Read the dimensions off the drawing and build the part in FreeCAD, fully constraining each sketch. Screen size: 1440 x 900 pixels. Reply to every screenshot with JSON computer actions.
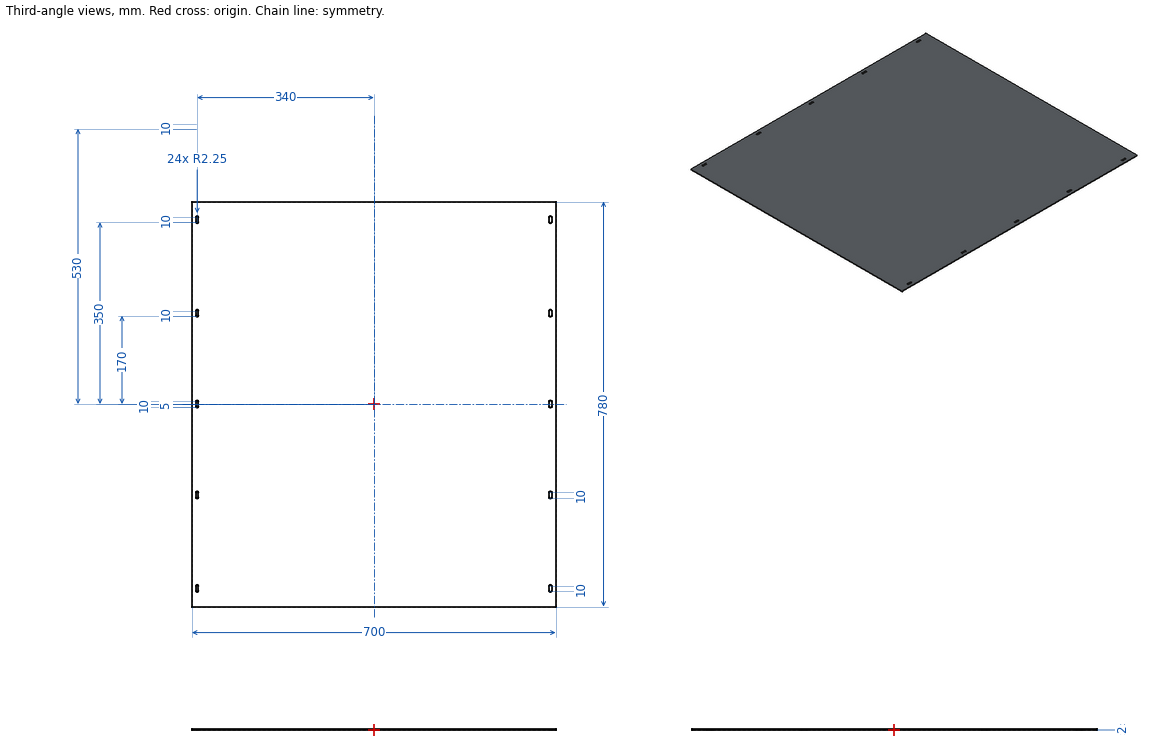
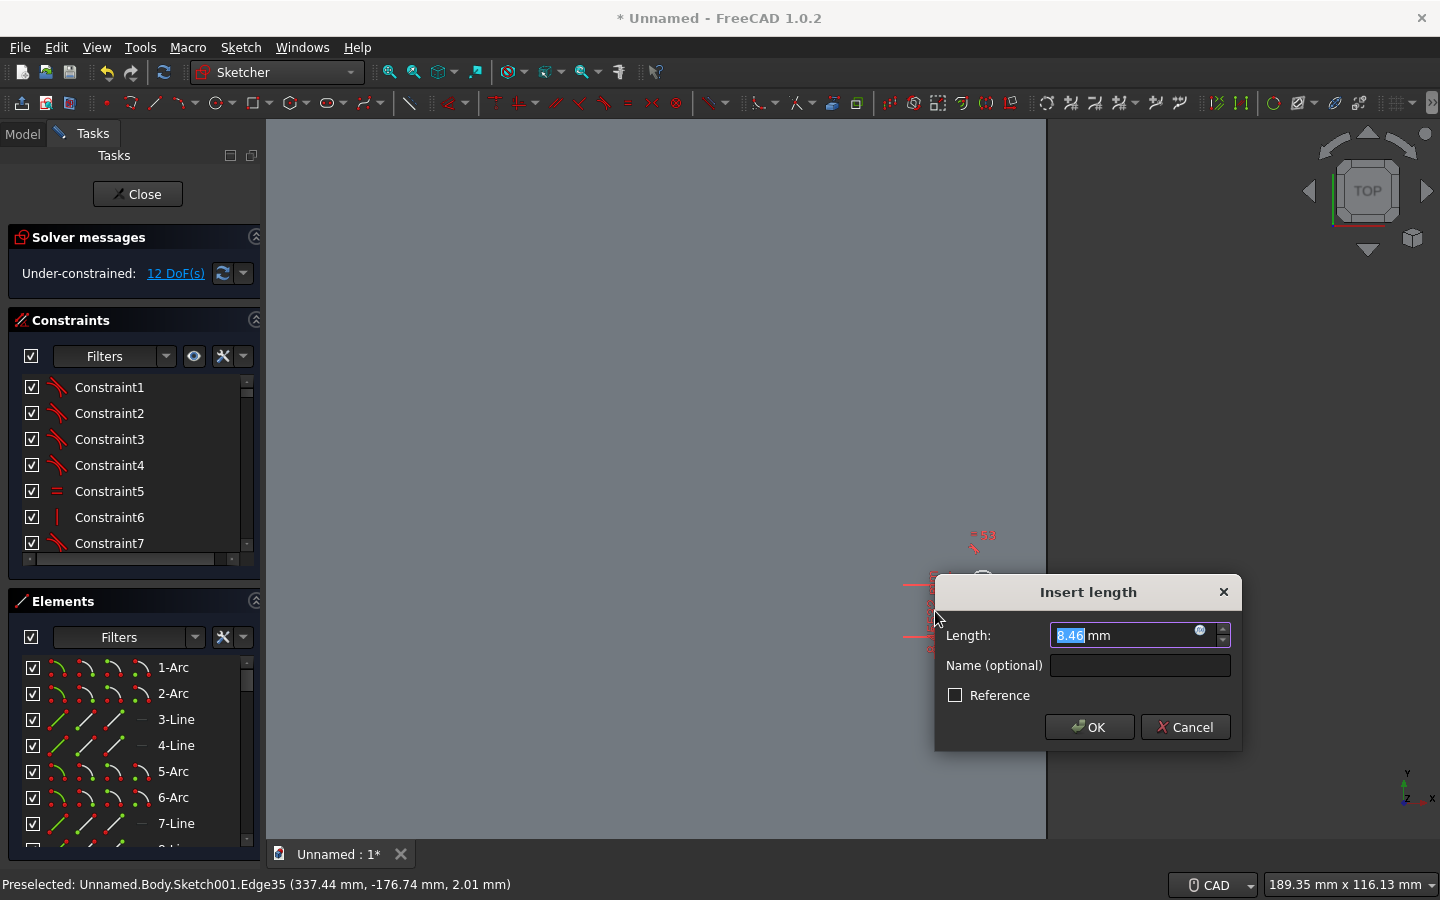
{"action": "type", "text": "10"}
{"action": "key", "text": "Return"}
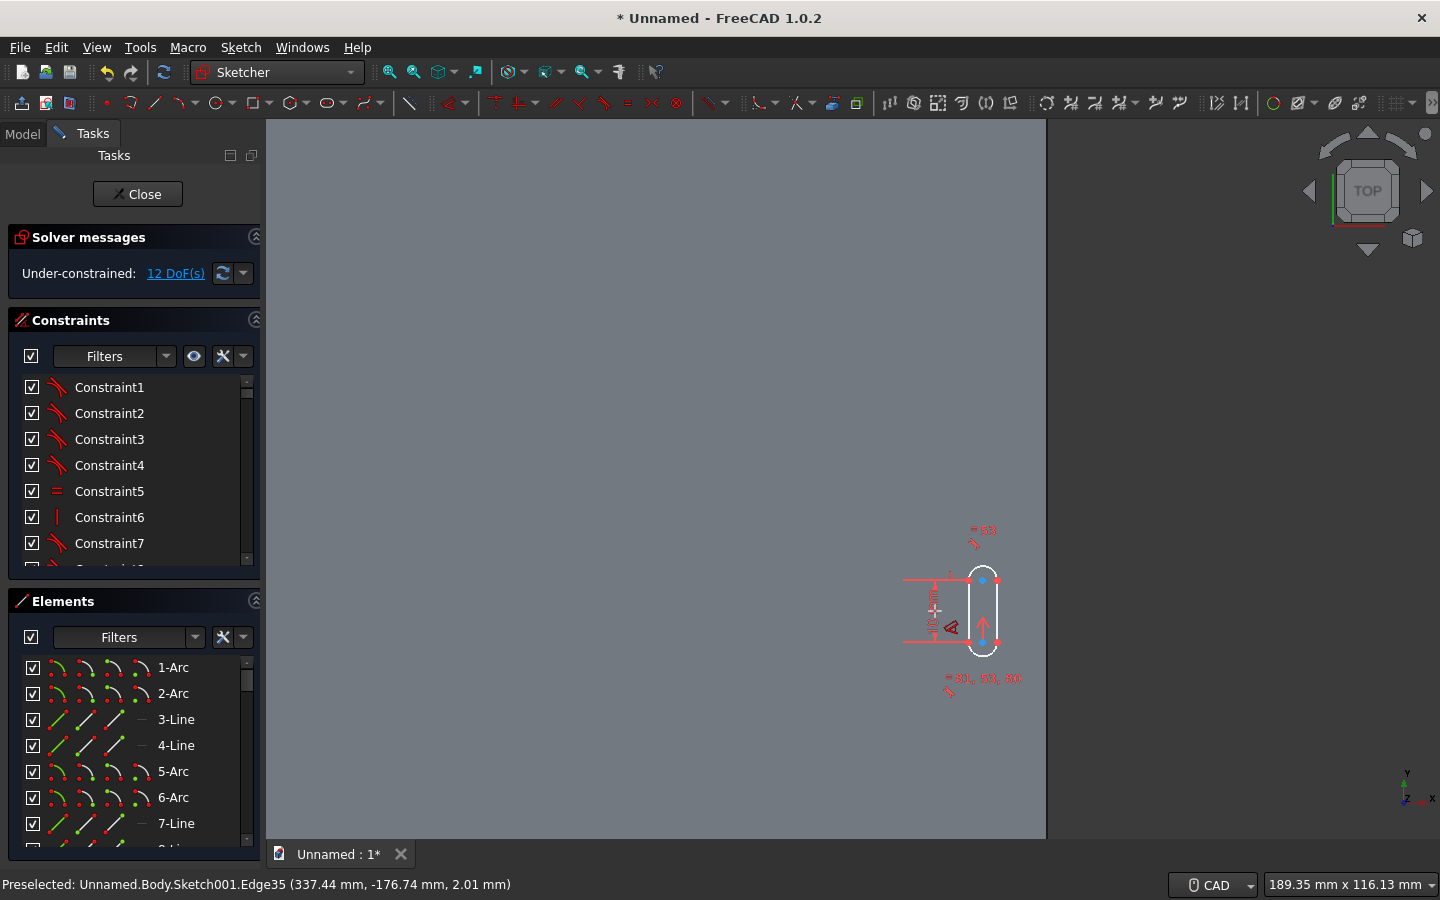
{"action": "scroll", "coordinate": [975, 630], "scroll_direction": "down", "scroll_amount": 12}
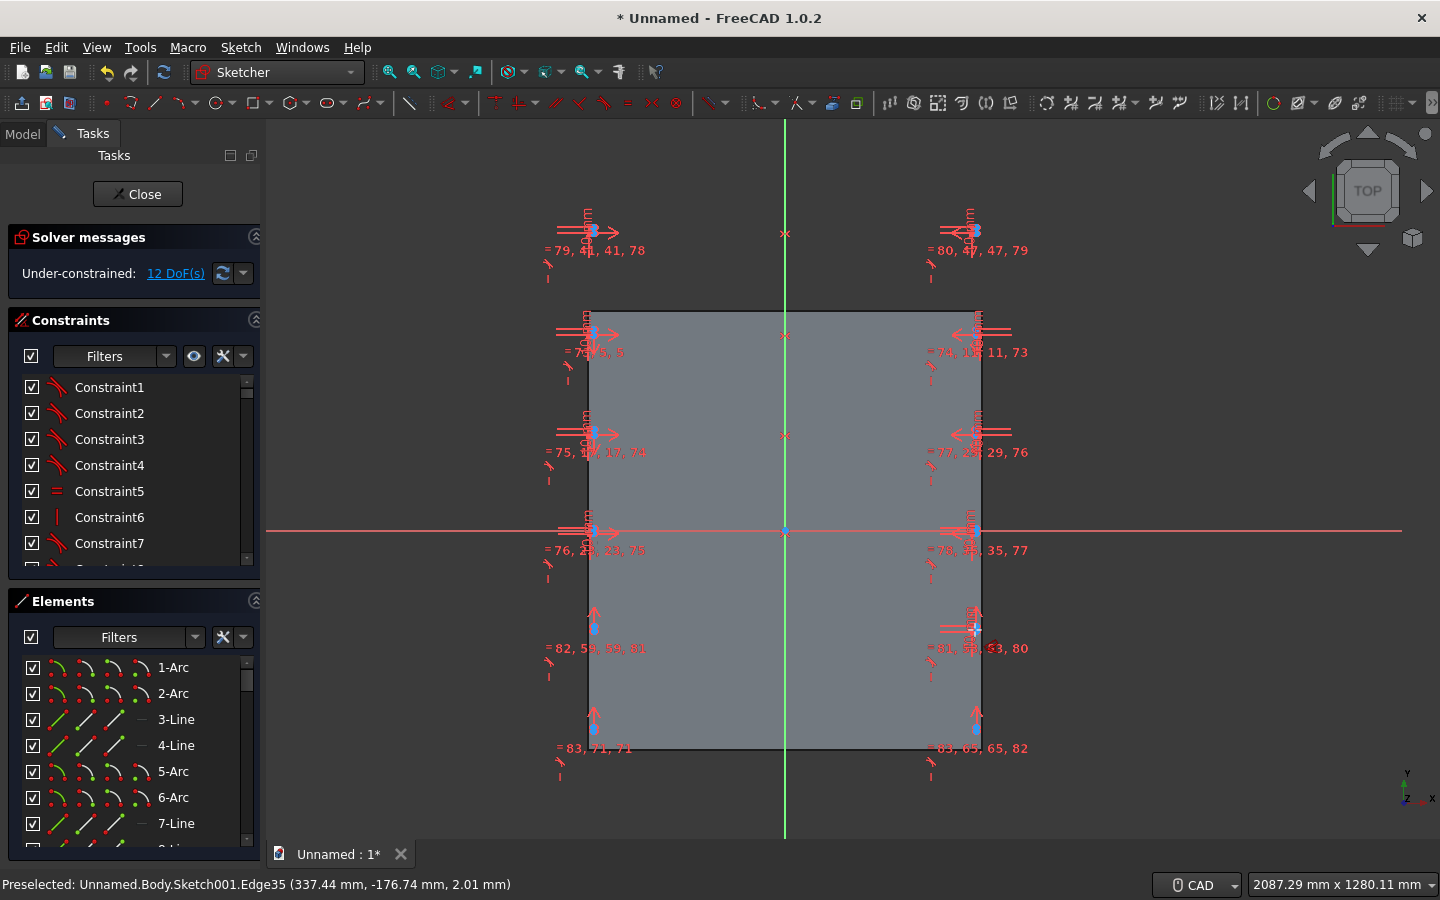
{"action": "scroll", "coordinate": [593, 630], "scroll_direction": "up", "scroll_amount": 11}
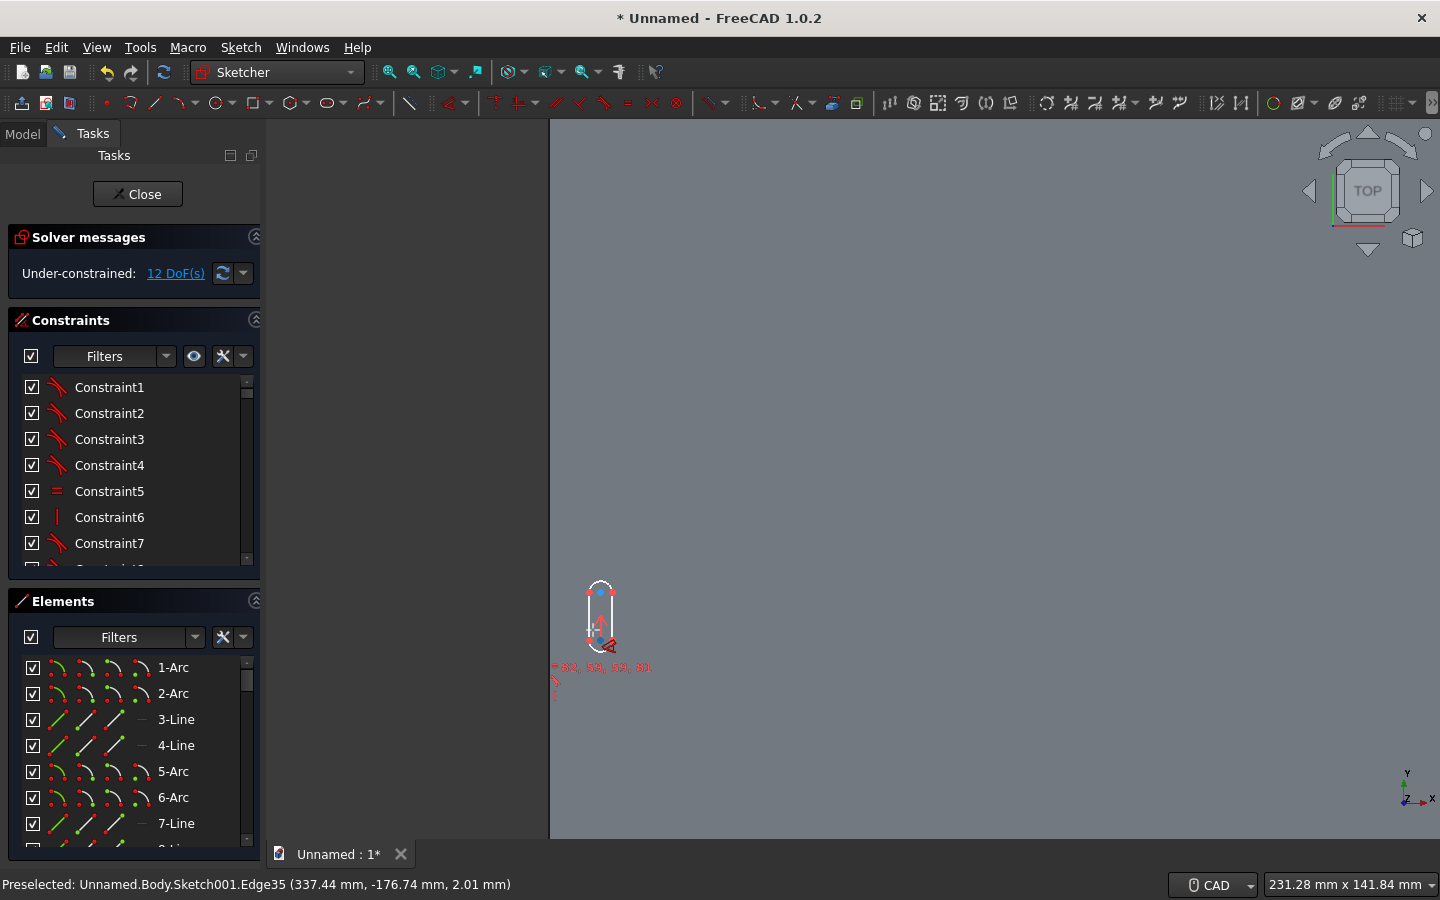
{"action": "left_click", "coordinate": [589, 626]}
{"action": "left_click", "coordinate": [555, 617]}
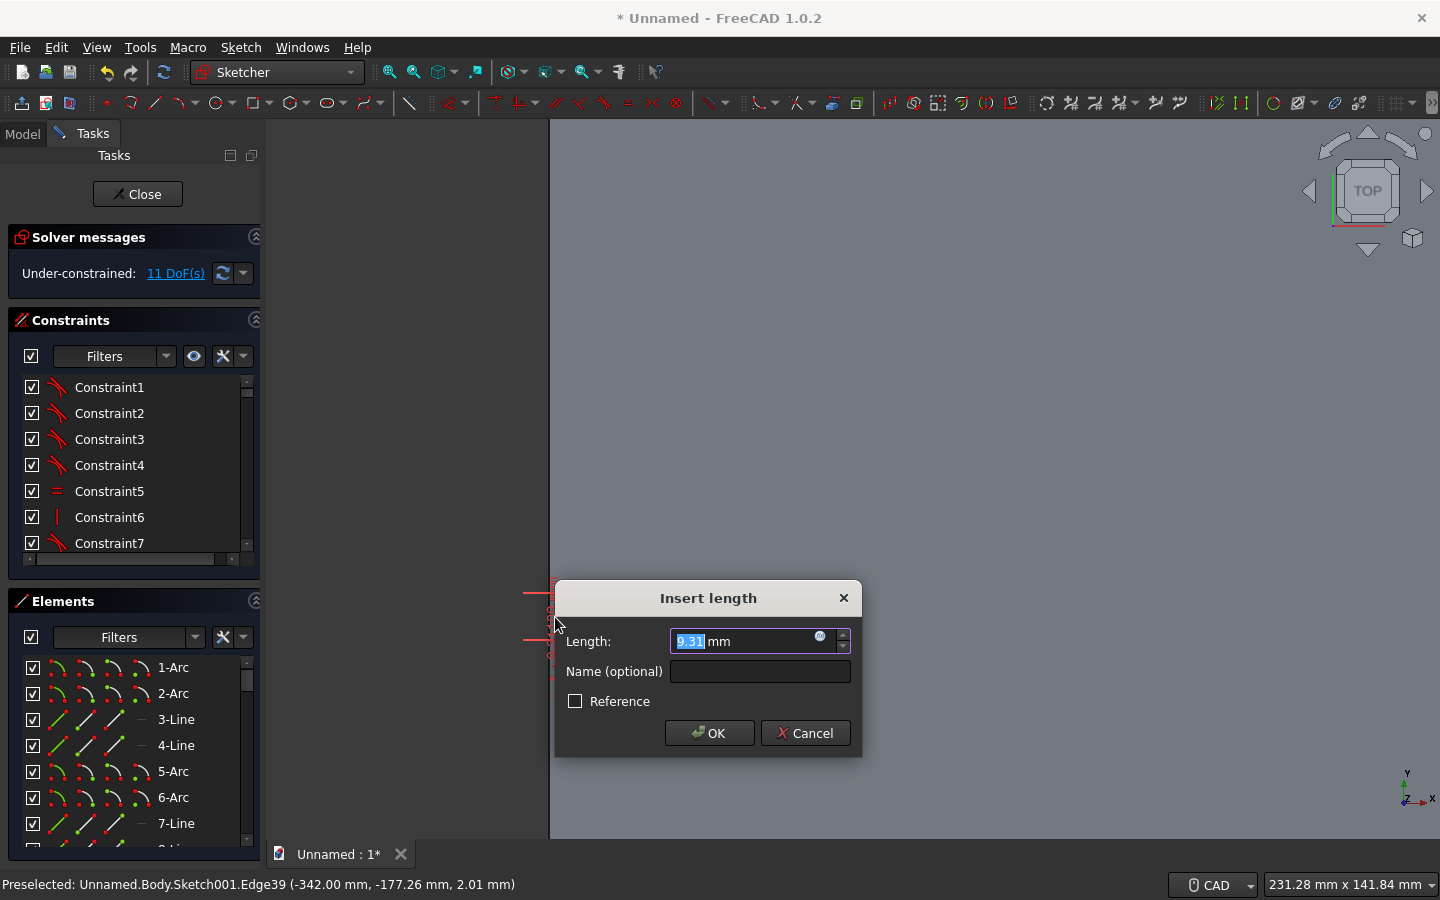
{"action": "type", "text": "10"}
{"action": "key", "text": "Return"}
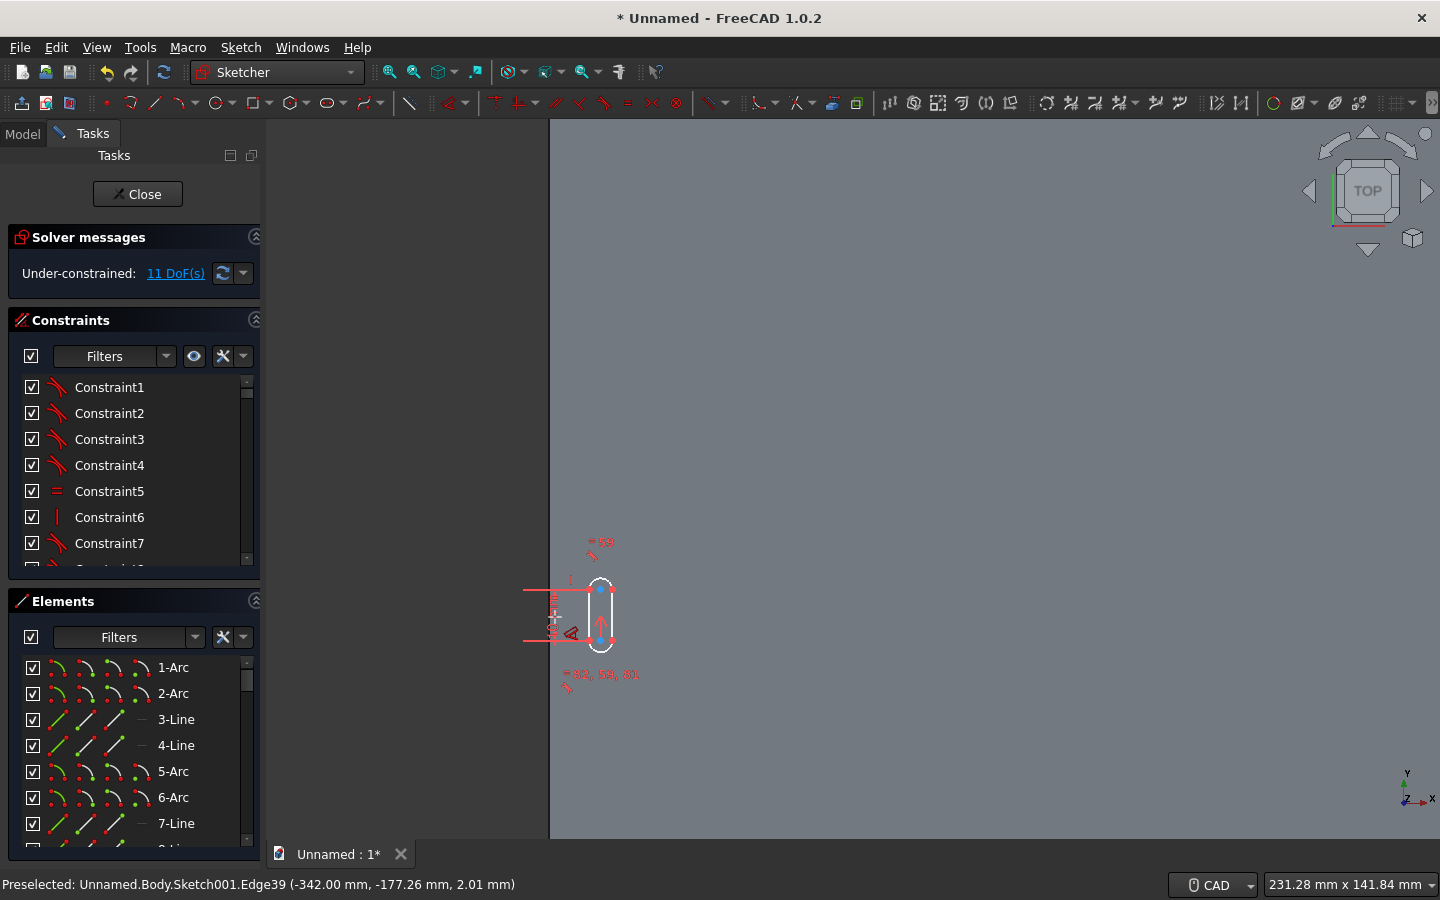
{"action": "scroll", "coordinate": [593, 630], "scroll_direction": "down", "scroll_amount": 11}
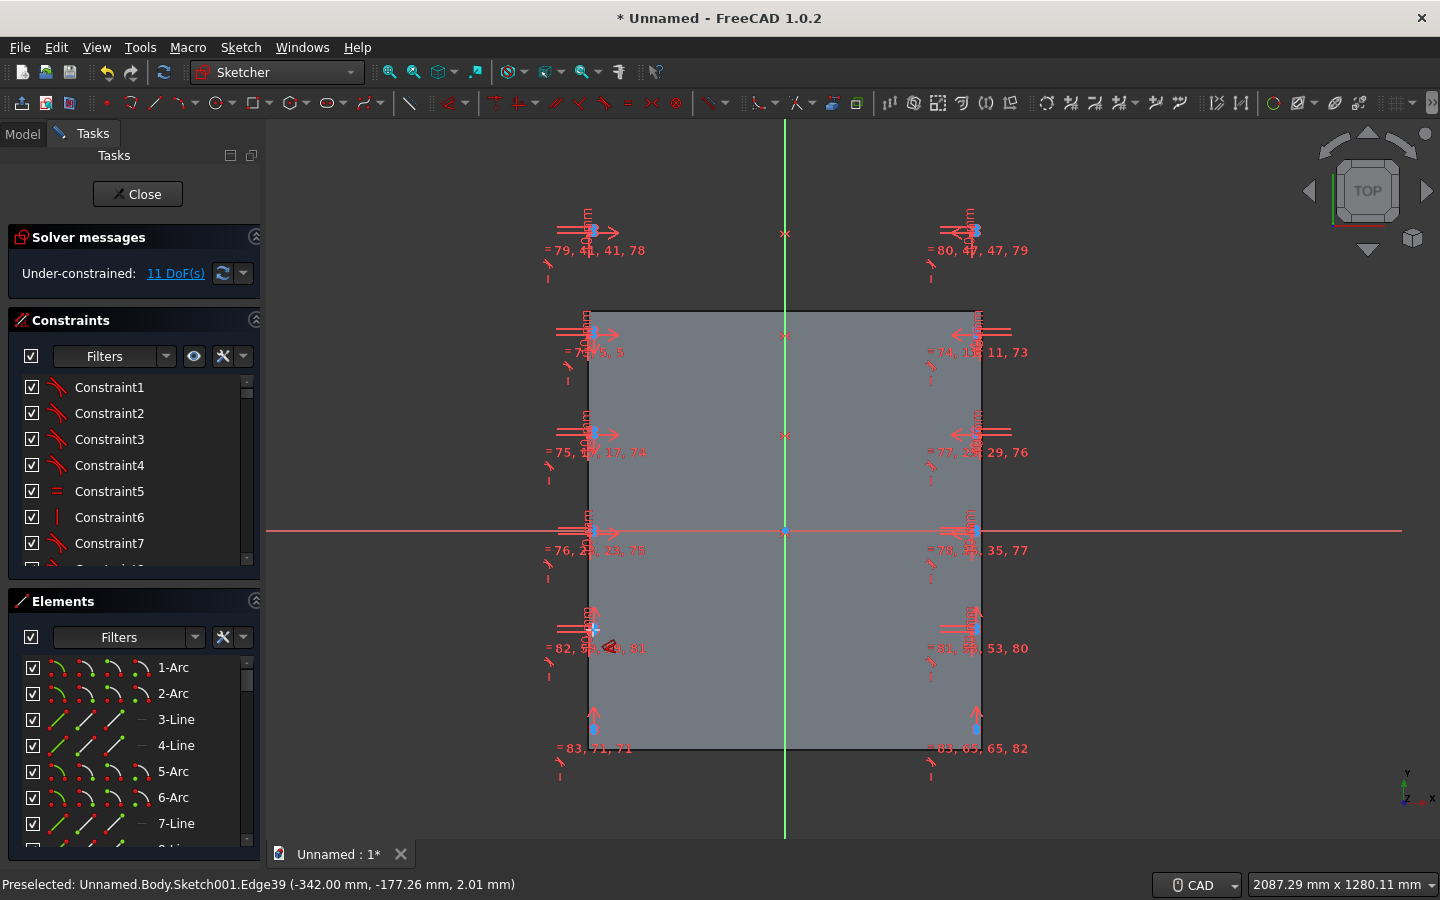
{"action": "scroll", "coordinate": [975, 731], "scroll_direction": "up", "scroll_amount": 13}